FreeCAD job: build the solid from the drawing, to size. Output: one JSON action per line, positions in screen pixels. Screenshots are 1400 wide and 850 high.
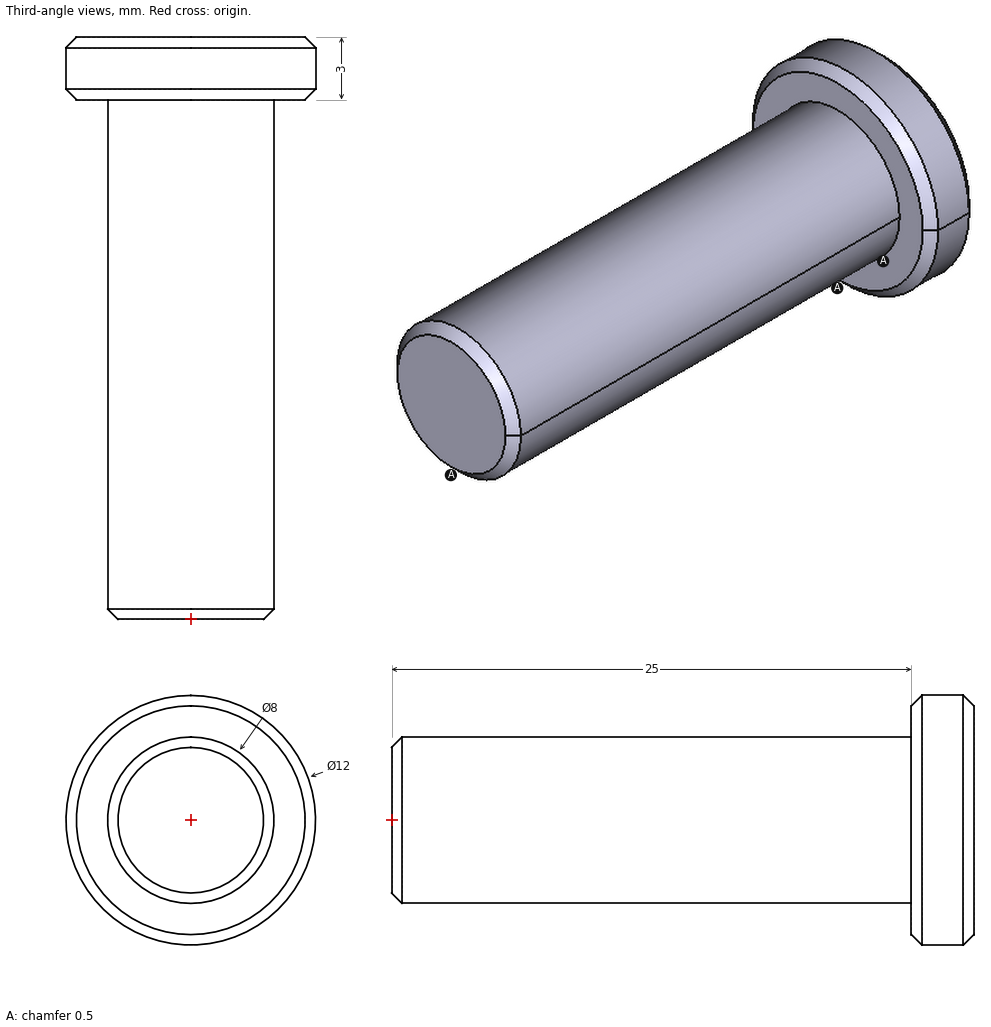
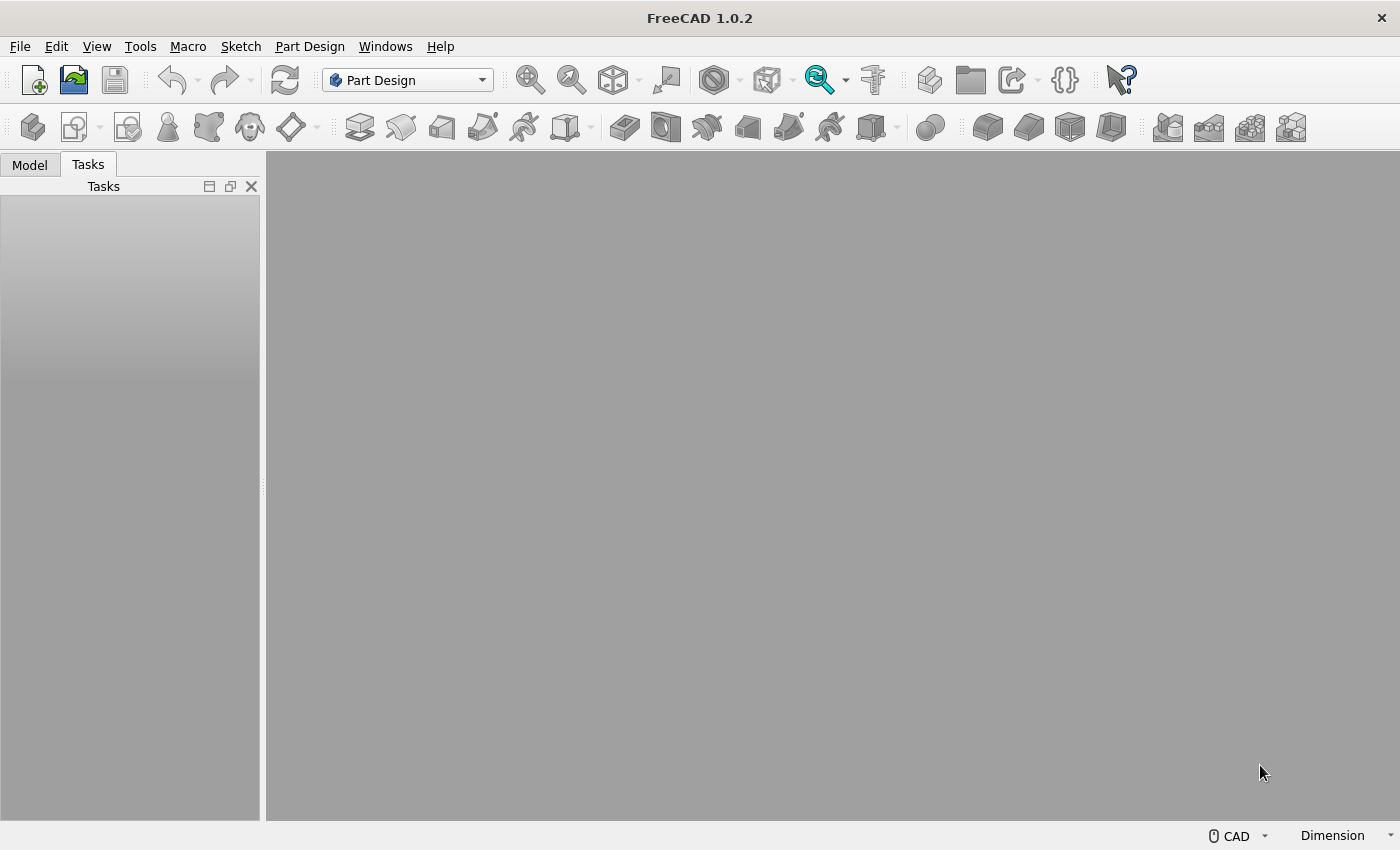
{"action": "key", "text": "ctrl+n"}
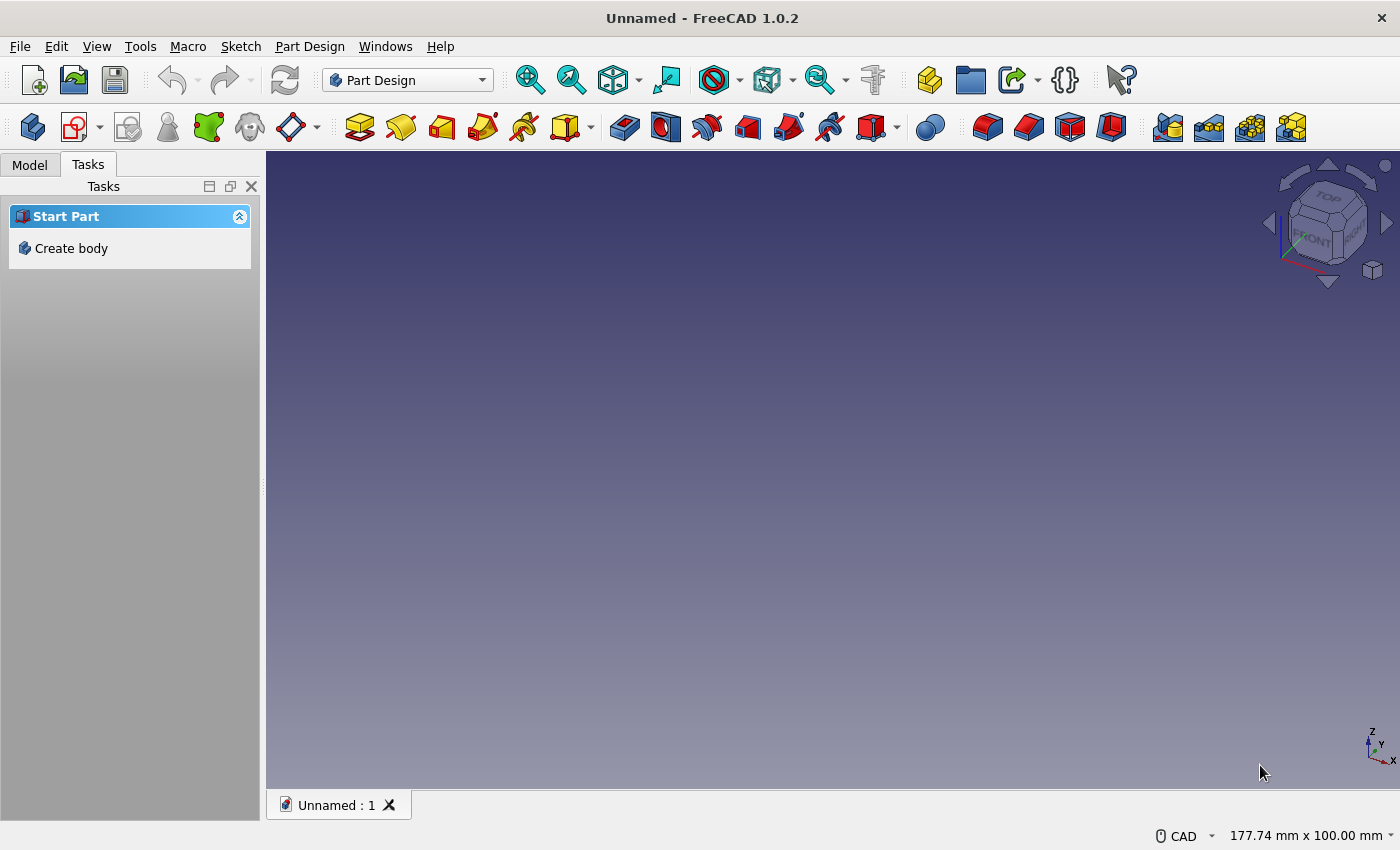
{"action": "left_click", "coordinate": [74, 128]}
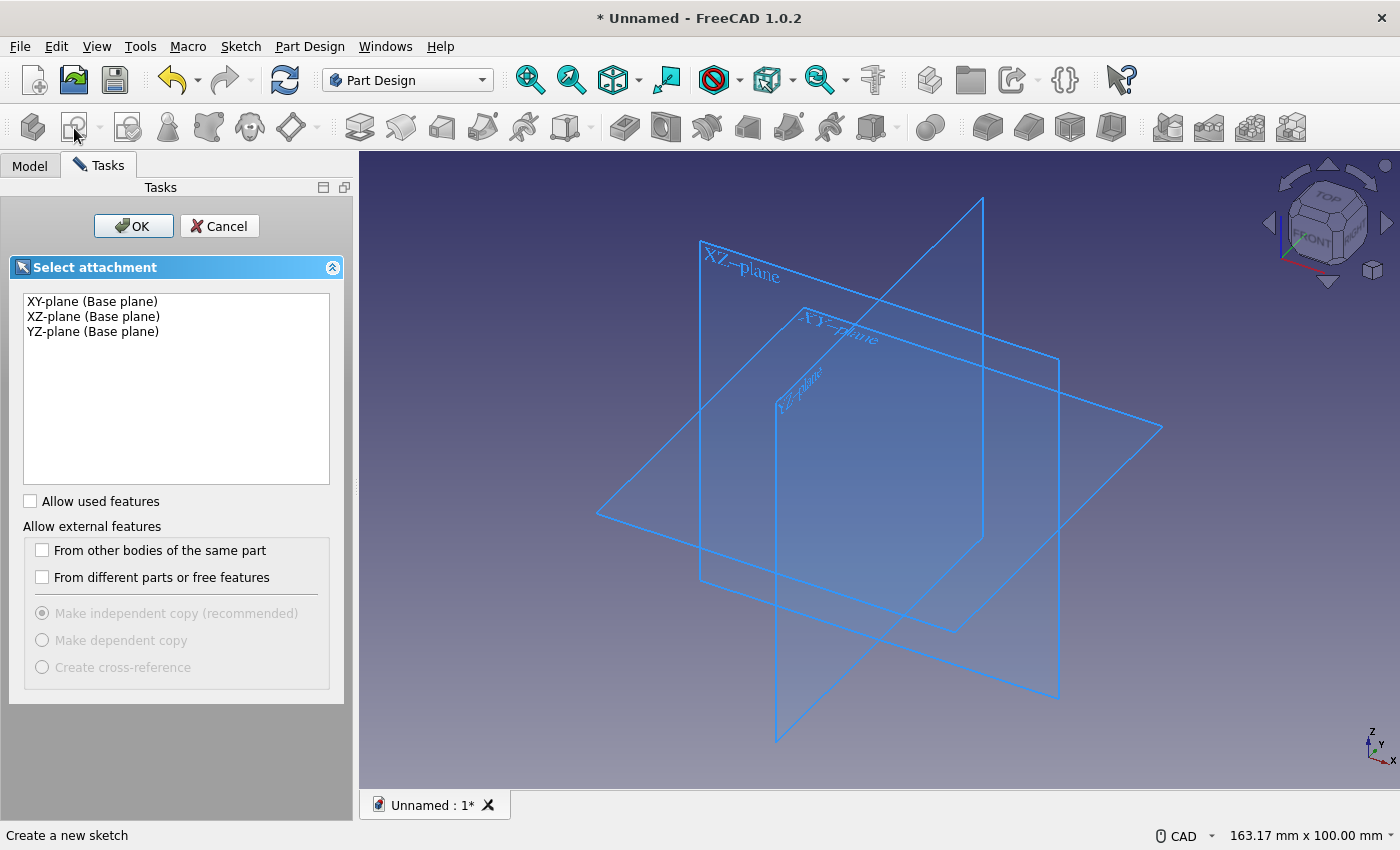
{"action": "left_click", "coordinate": [84, 316]}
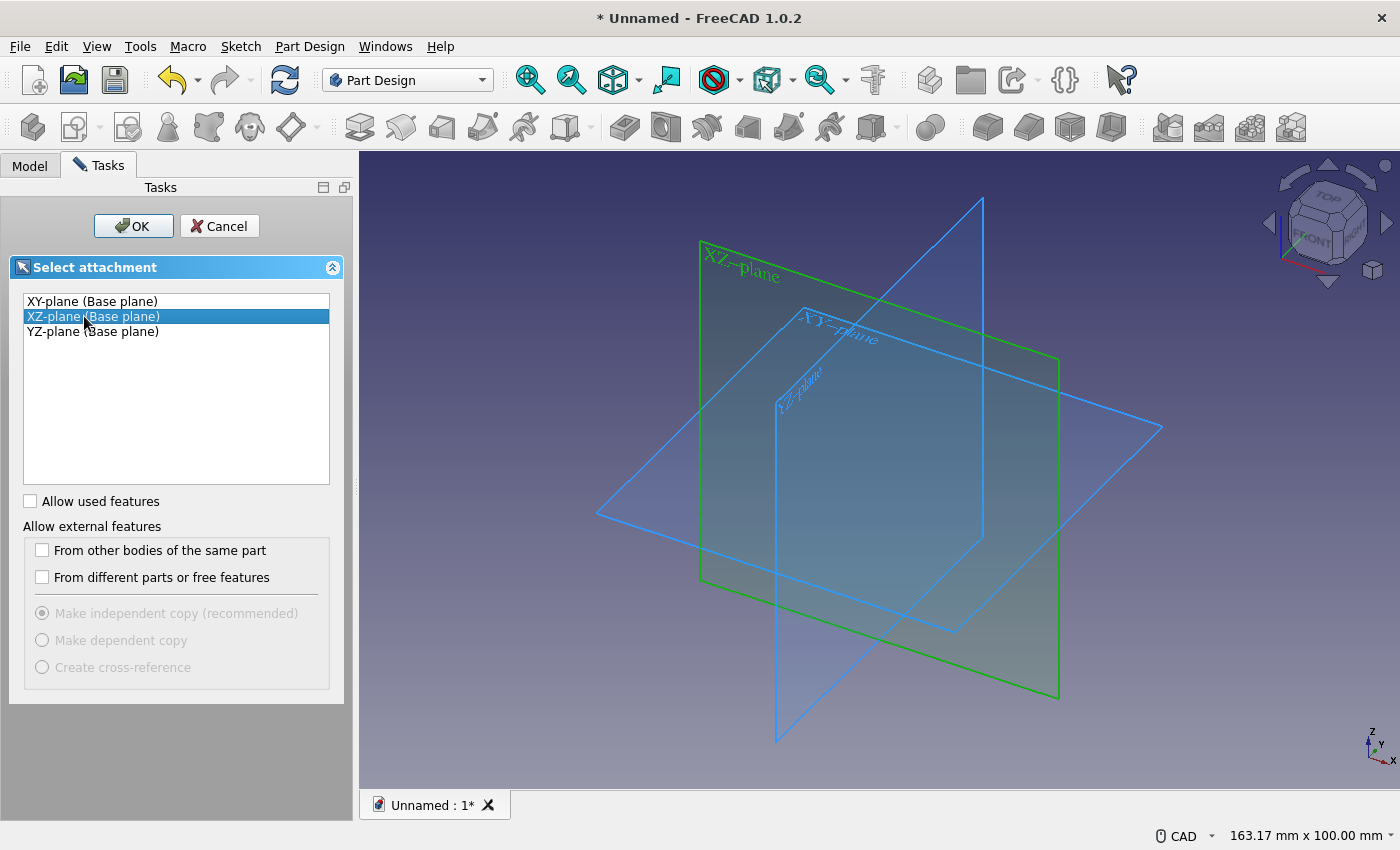
{"action": "left_click", "coordinate": [134, 226]}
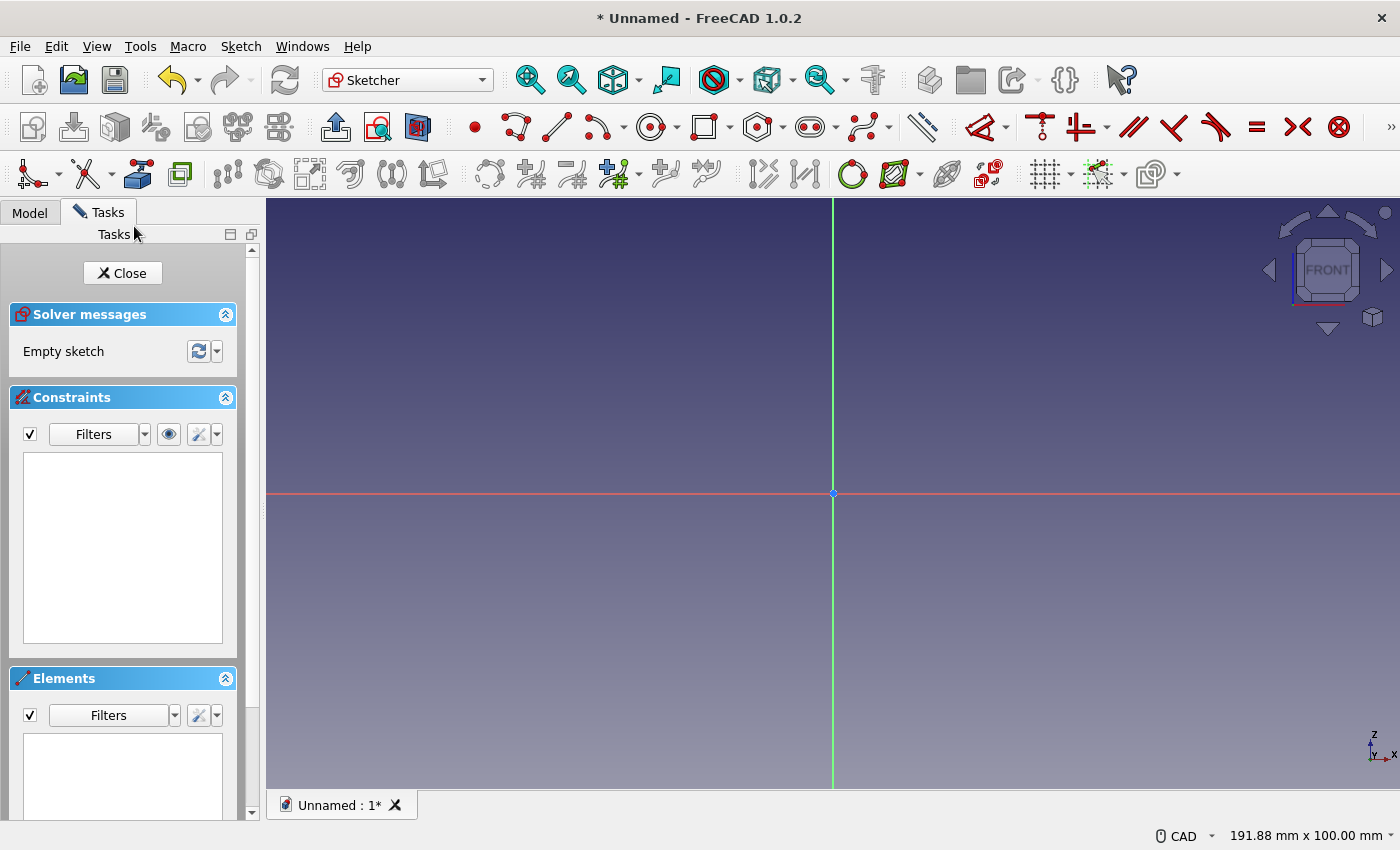
{"action": "scroll", "coordinate": [844, 493], "scroll_direction": "up", "scroll_amount": 10}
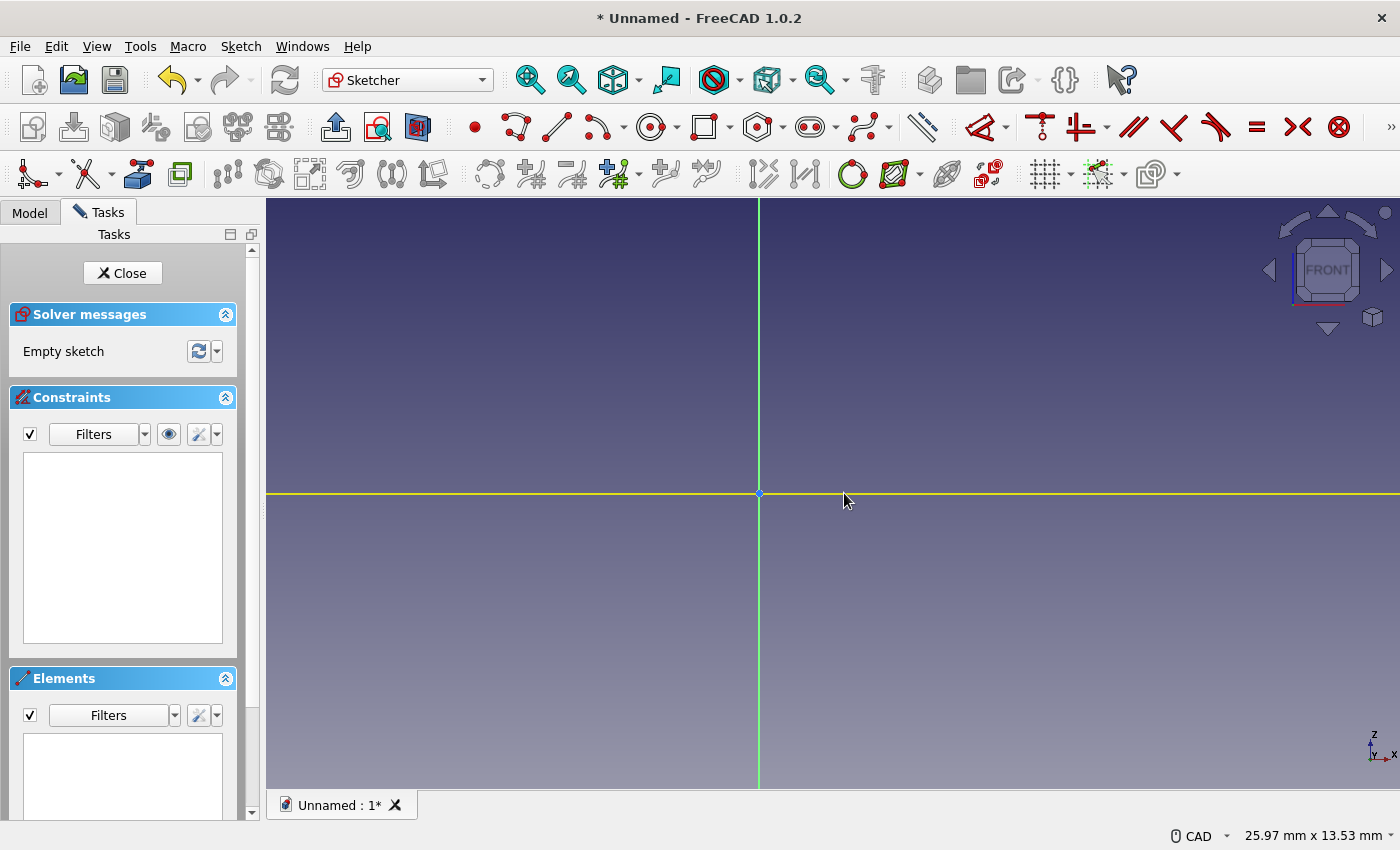
{"action": "key", "text": "g c"}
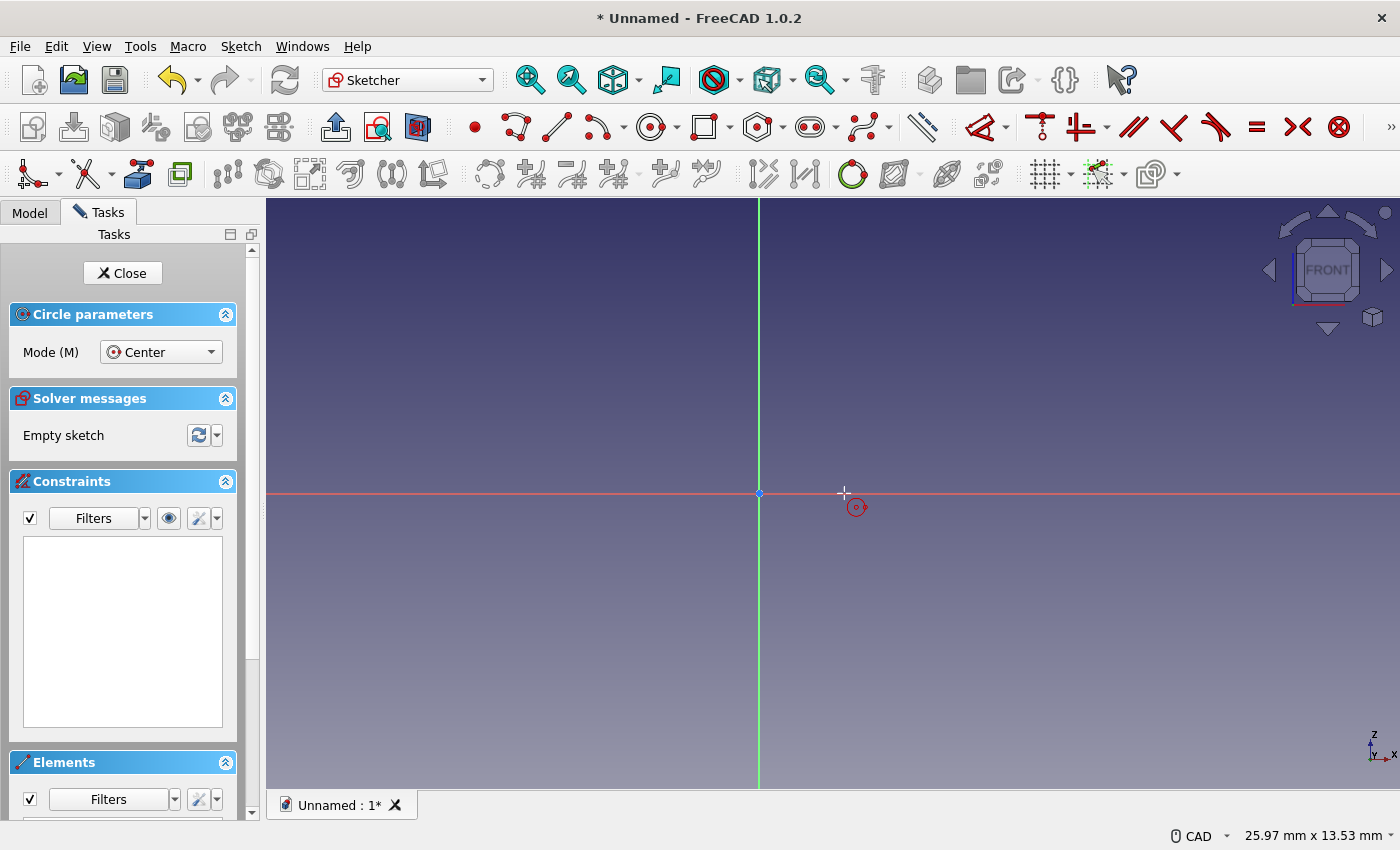
{"action": "left_click", "coordinate": [759, 494]}
{"action": "mouse_move", "coordinate": [883, 370]}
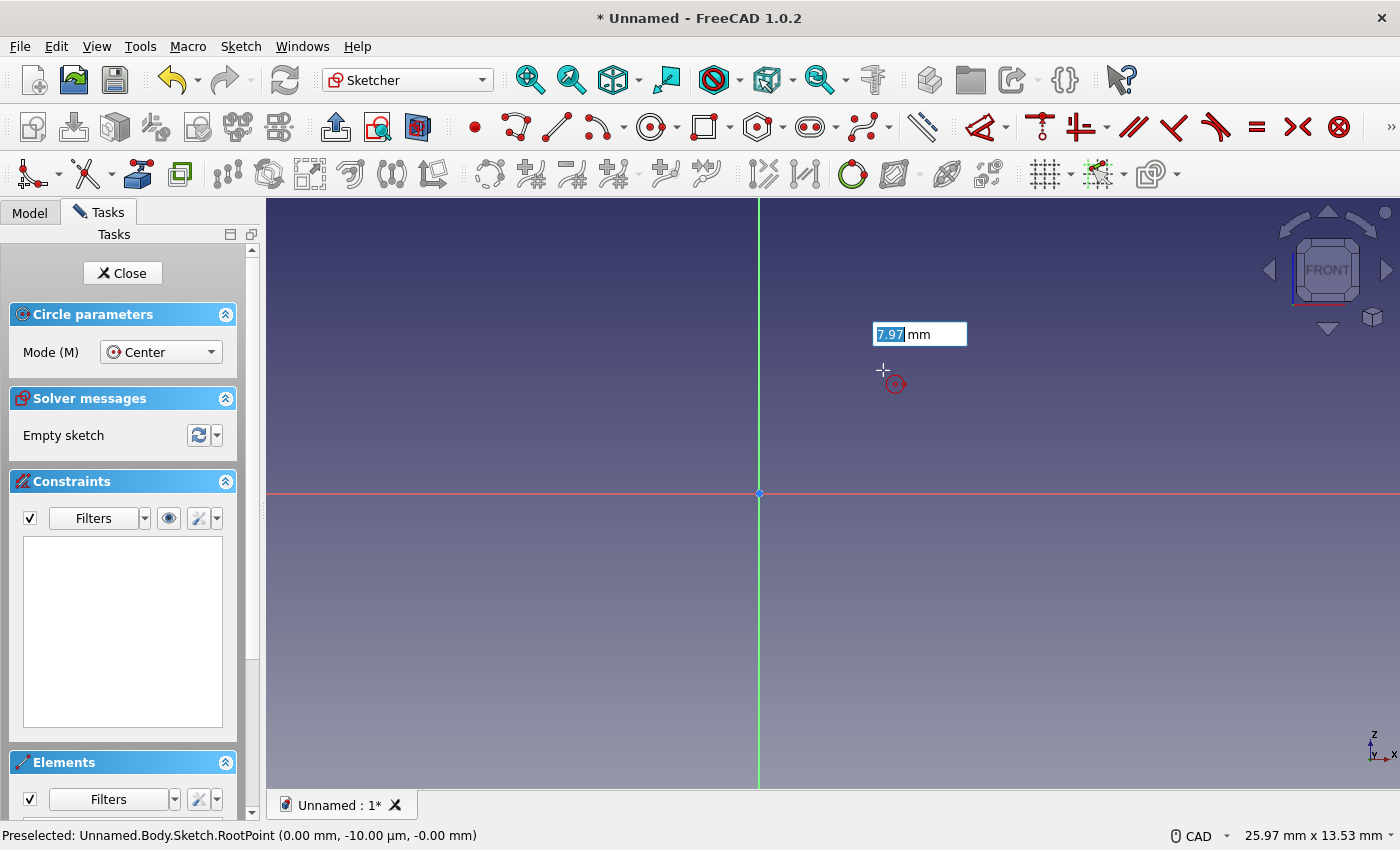
{"action": "type", "text": "8"}
{"action": "key", "text": "Return"}
{"action": "key", "text": "Escape"}